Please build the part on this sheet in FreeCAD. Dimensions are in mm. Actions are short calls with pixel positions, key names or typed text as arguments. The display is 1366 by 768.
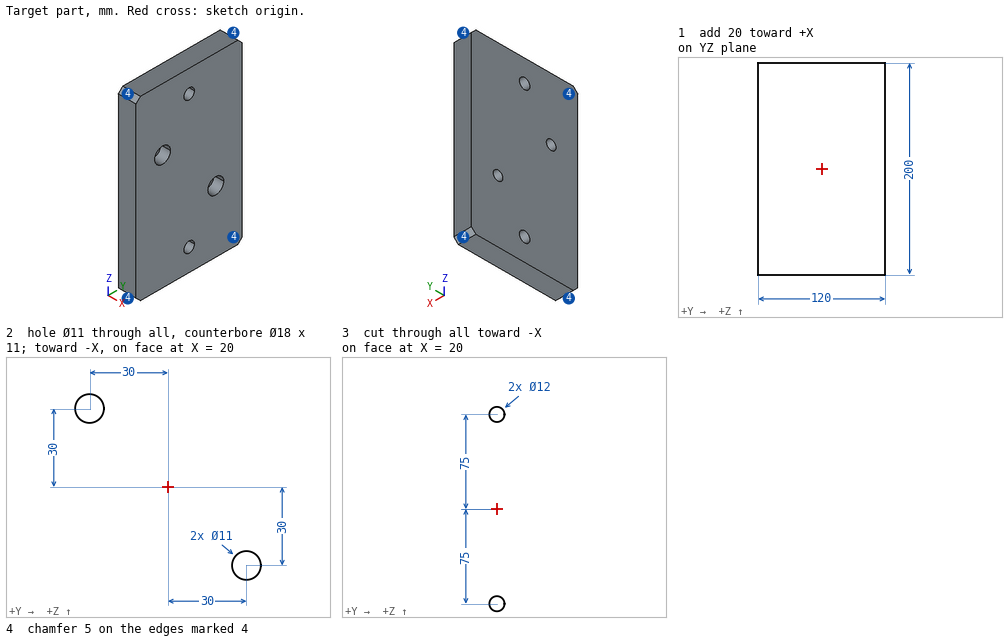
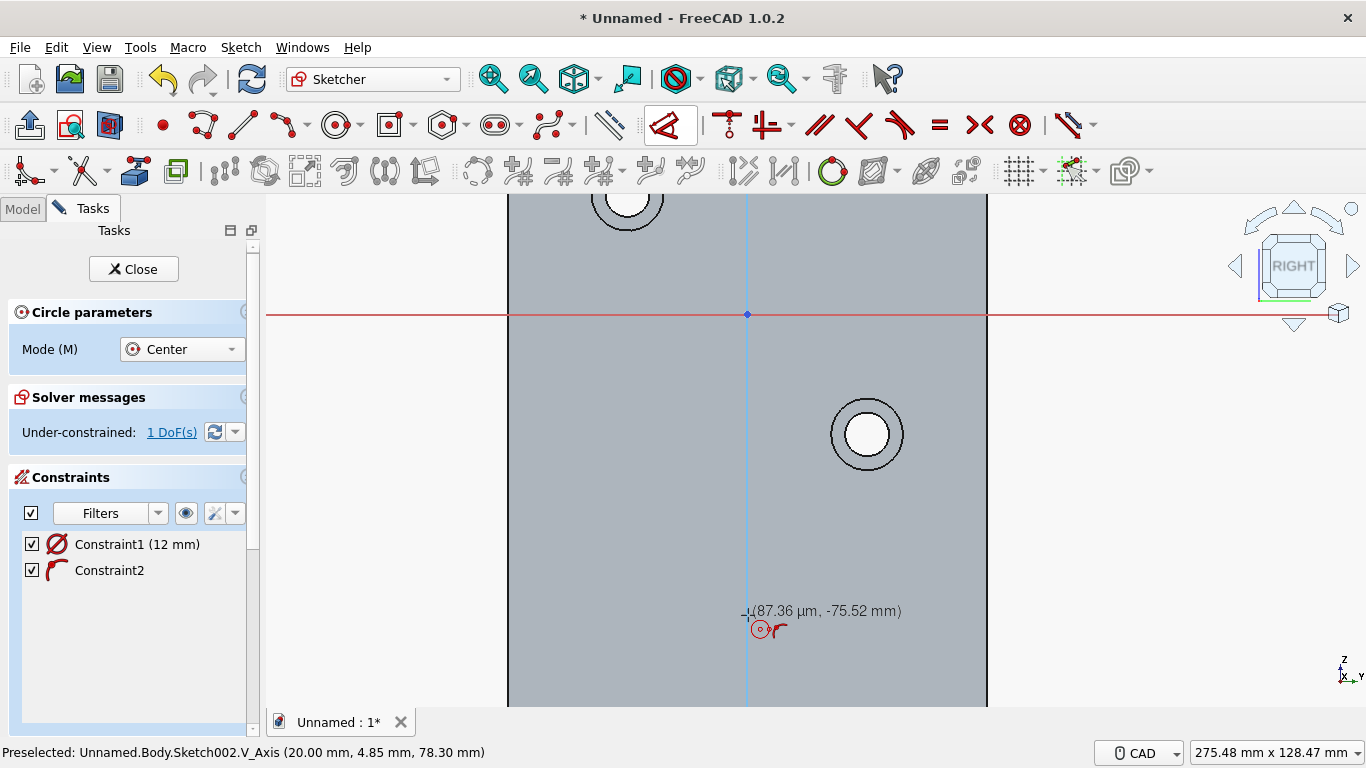
click(747, 614)
move(764, 597)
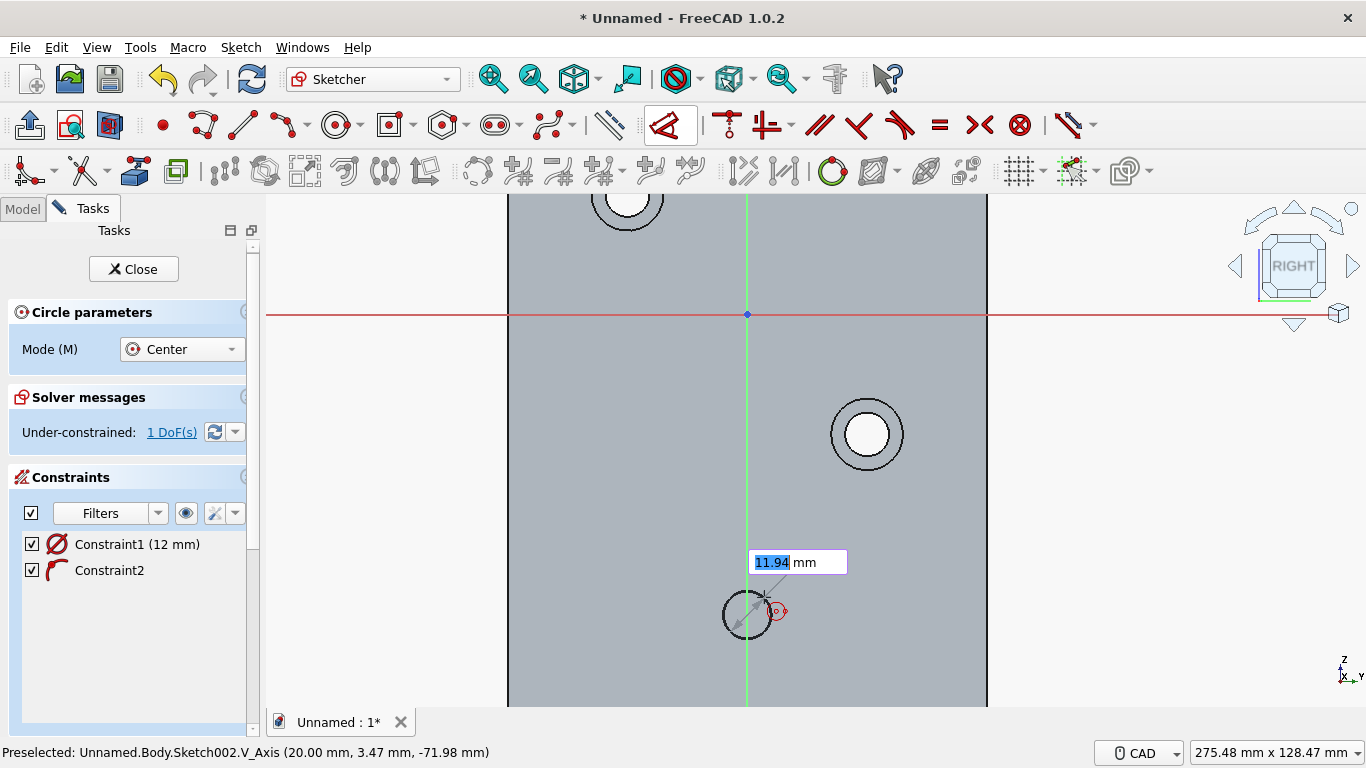
text(12)
key(Return)
key(Escape)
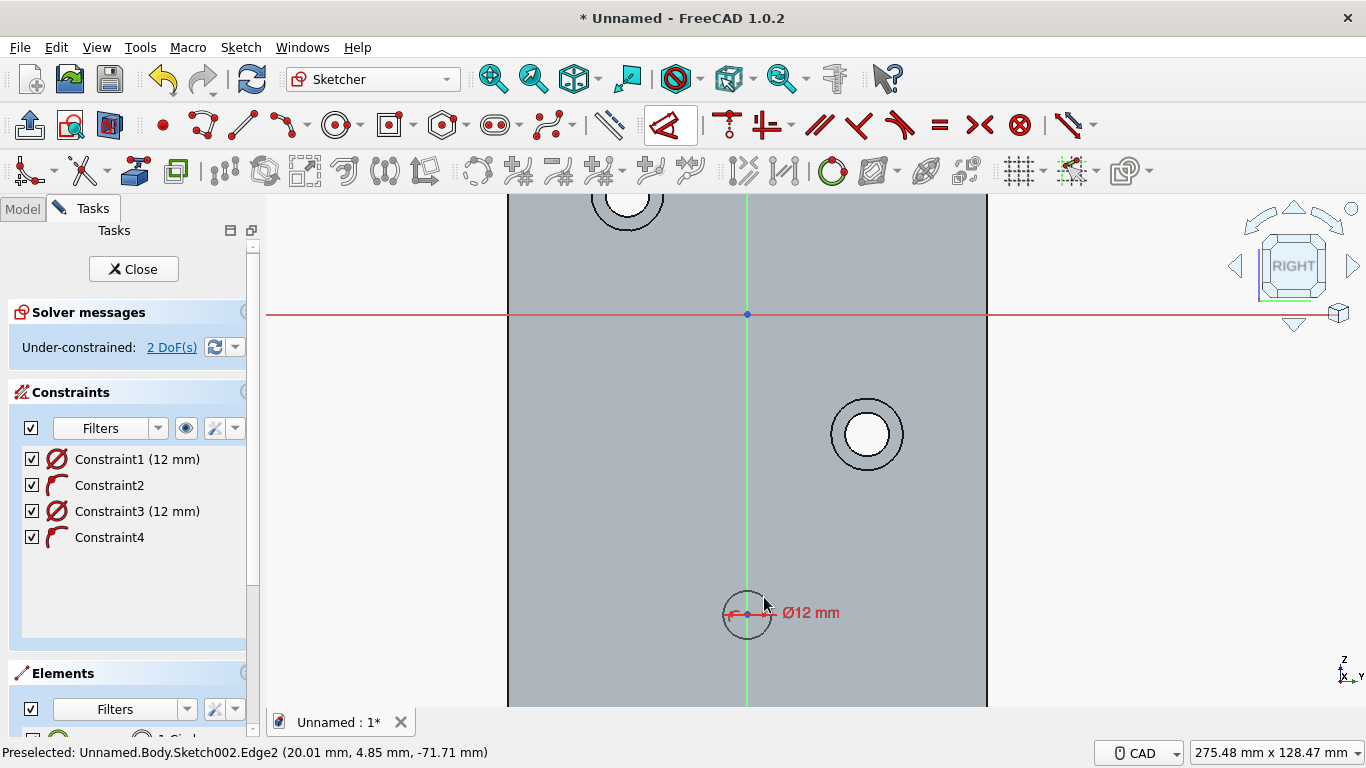
click(664, 126)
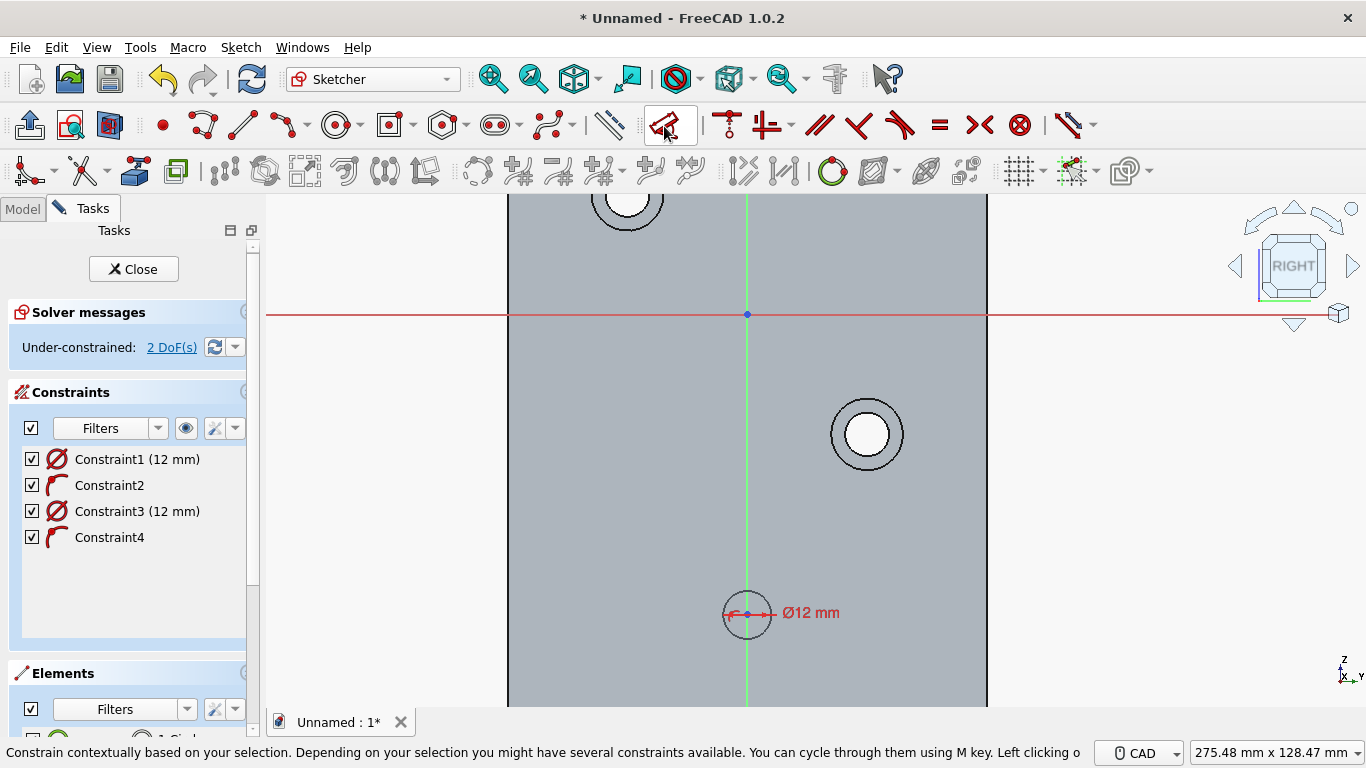
scroll(748, 616, down, 3)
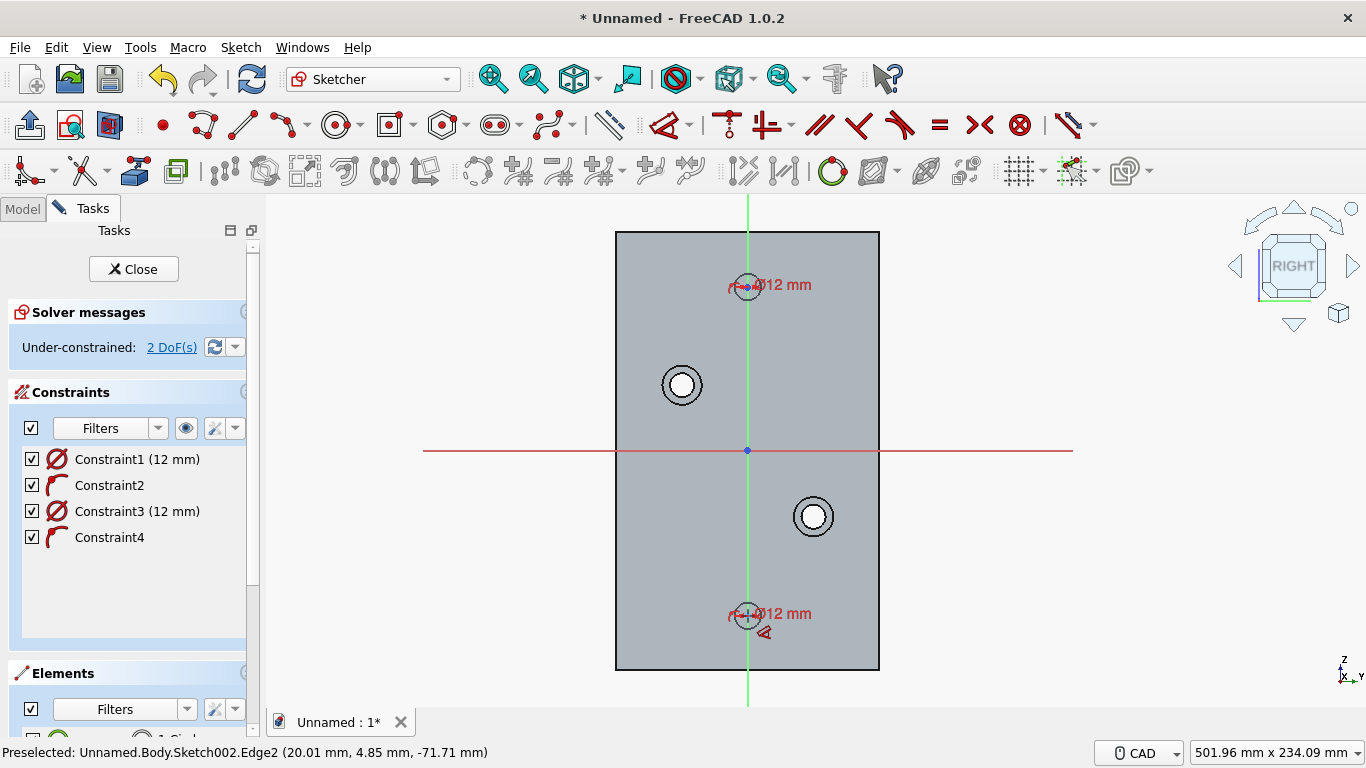
click(748, 287)
click(782, 369)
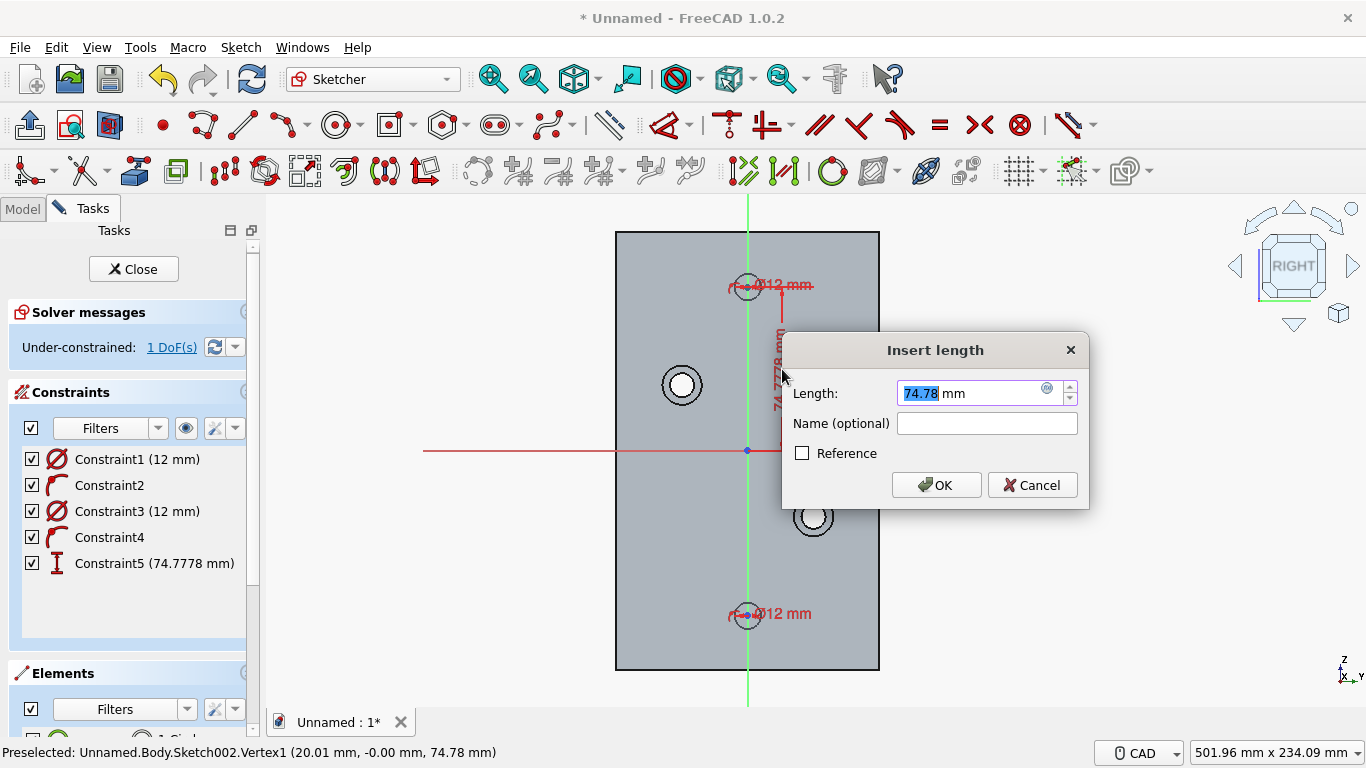
text(75)
key(Return)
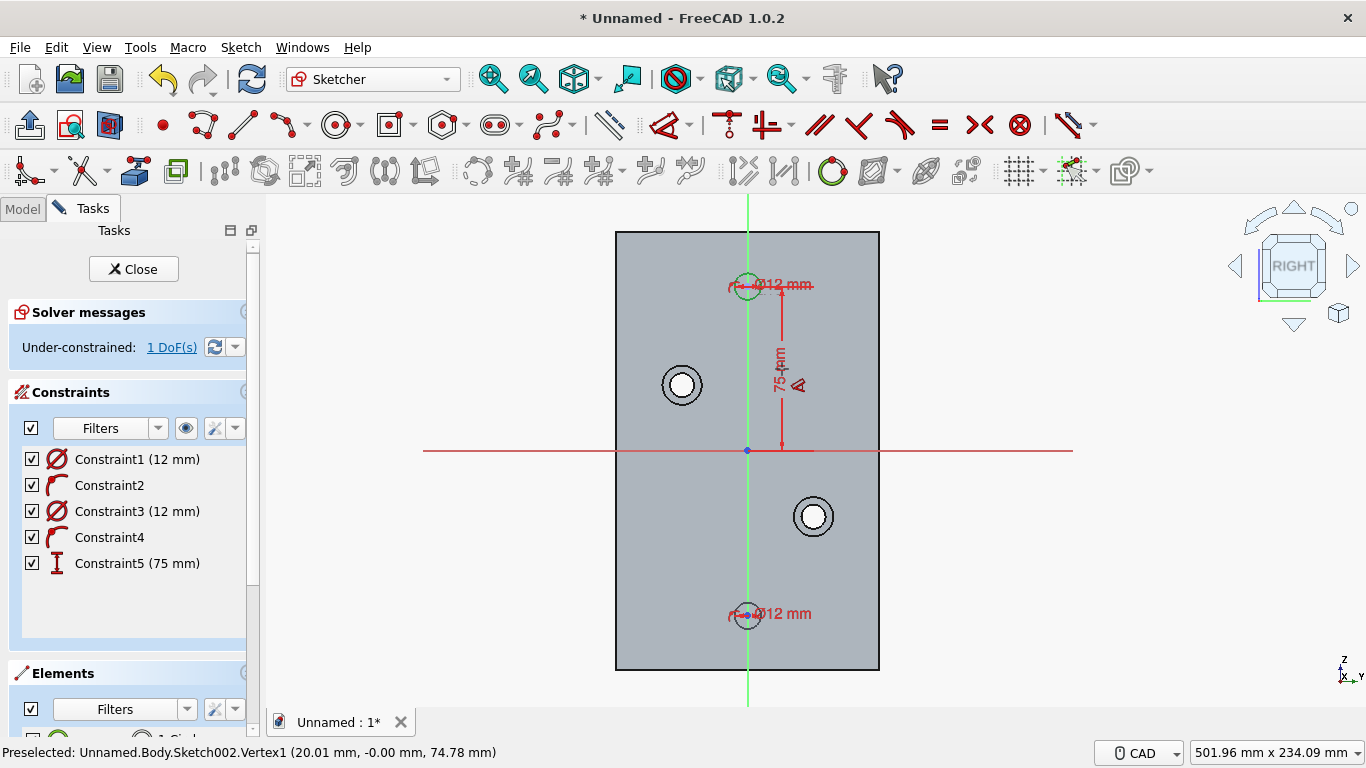
click(748, 616)
click(782, 533)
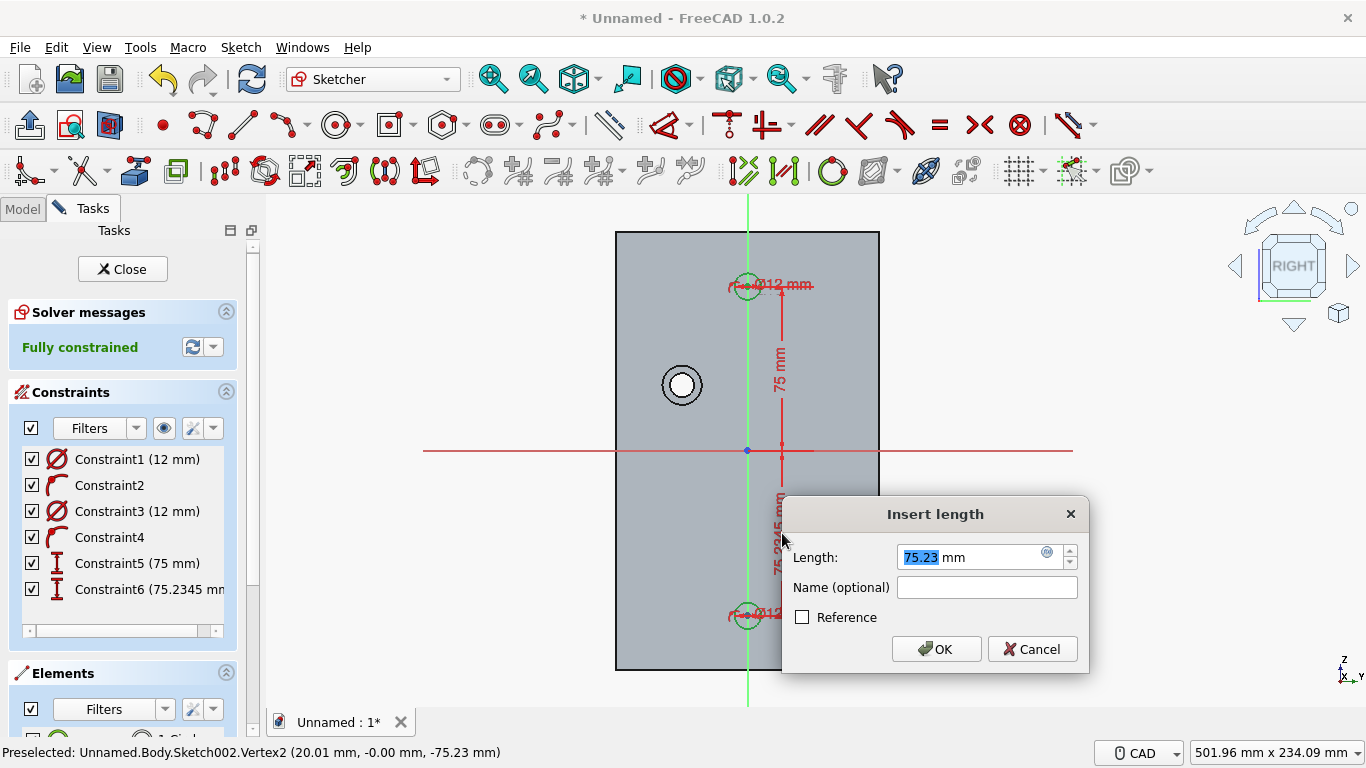
text(75)
key(Return)
key(Escape)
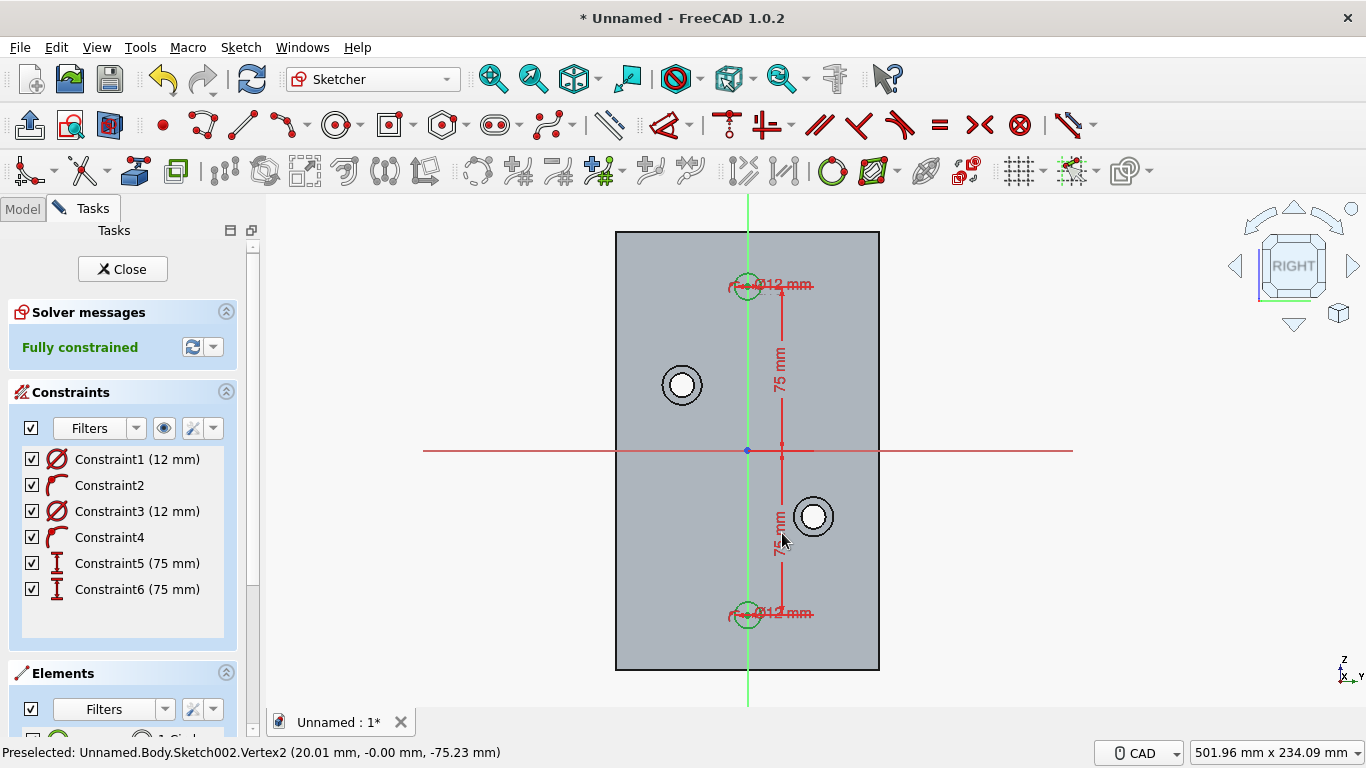
click(123, 269)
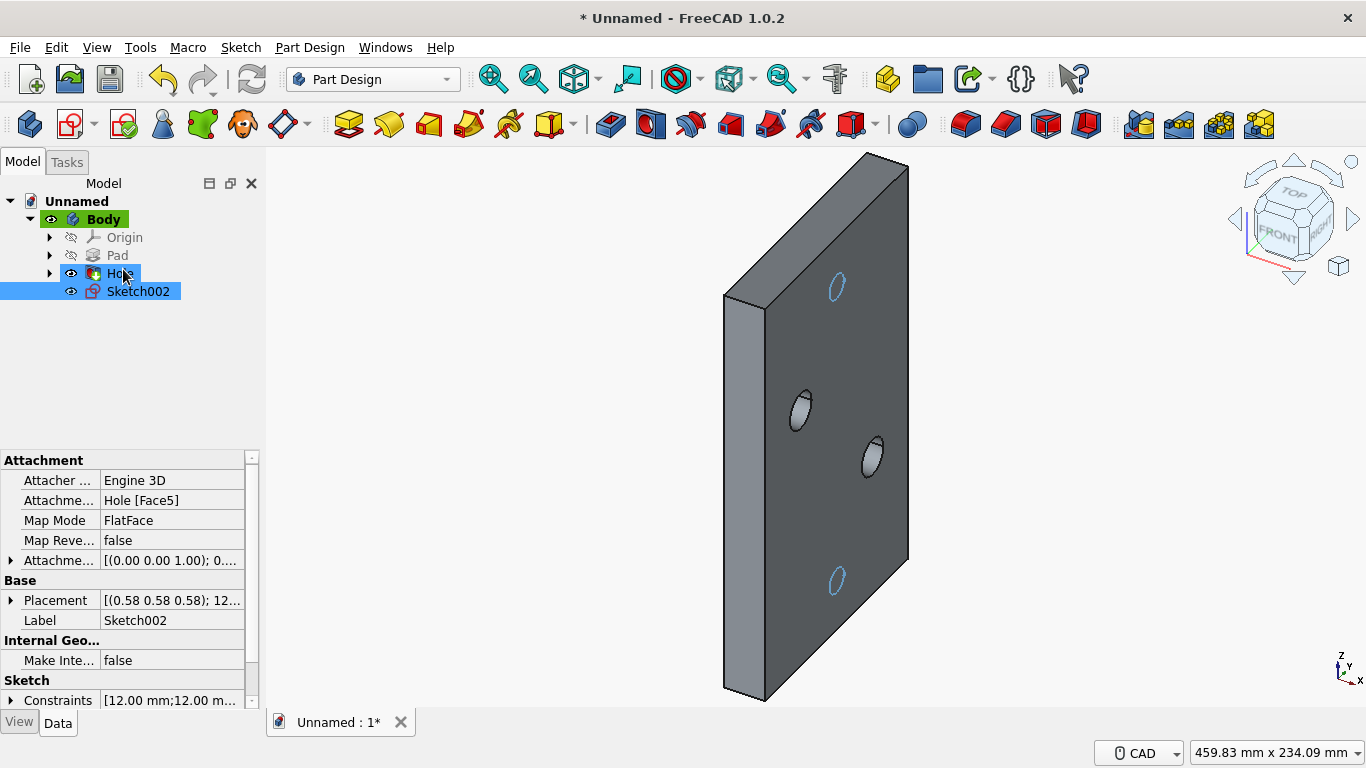
click(612, 124)